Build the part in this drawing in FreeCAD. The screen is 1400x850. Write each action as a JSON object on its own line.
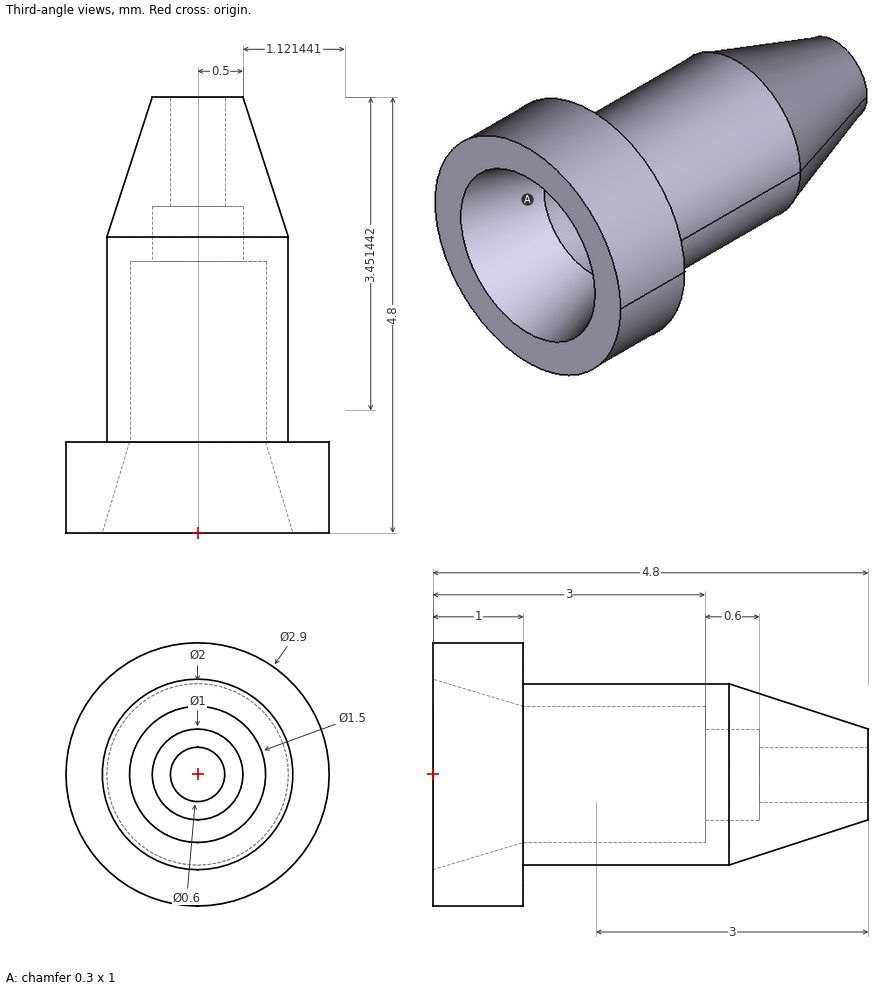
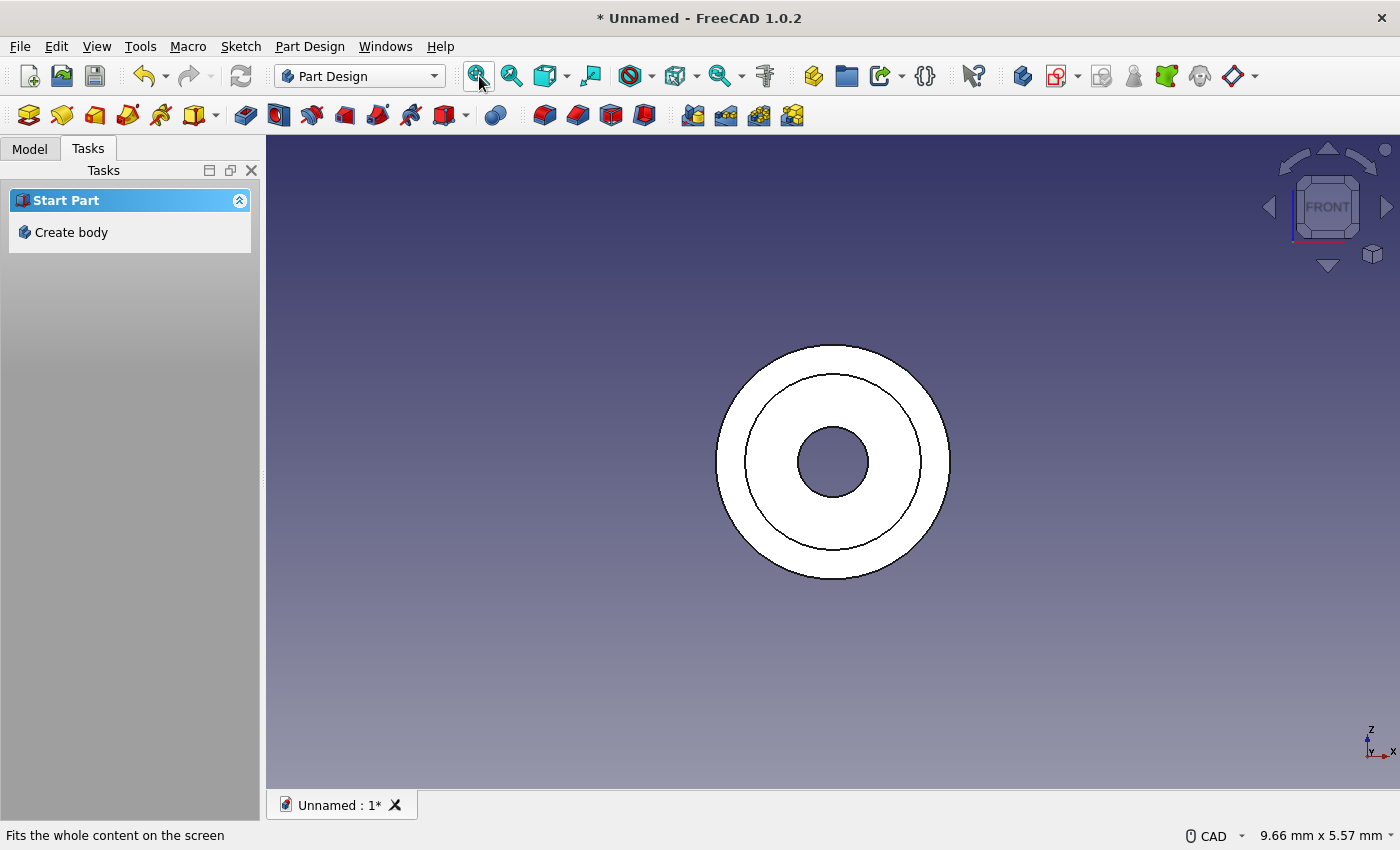
{"action": "left_click", "coordinate": [808, 511]}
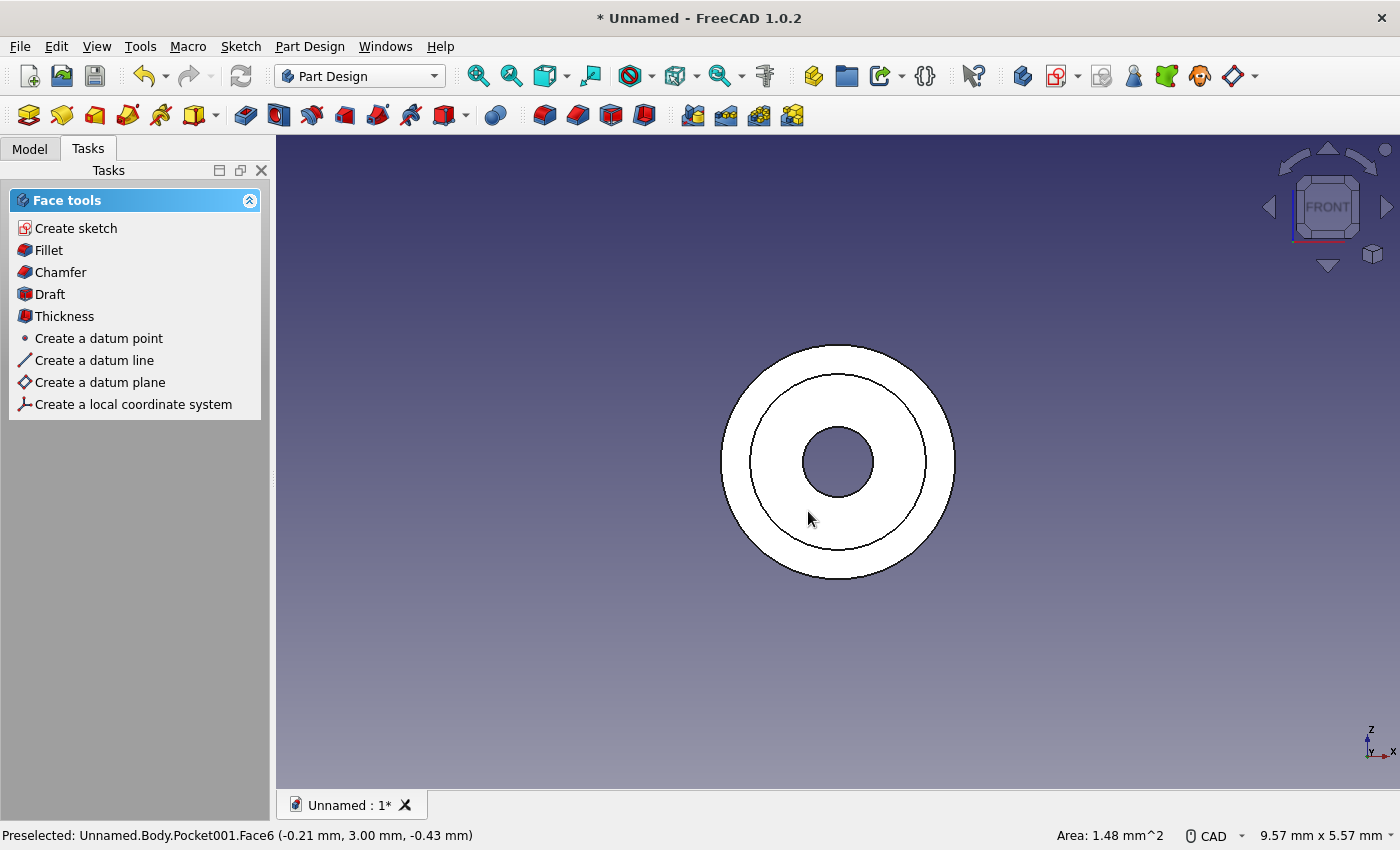
{"action": "left_click", "coordinate": [1056, 76]}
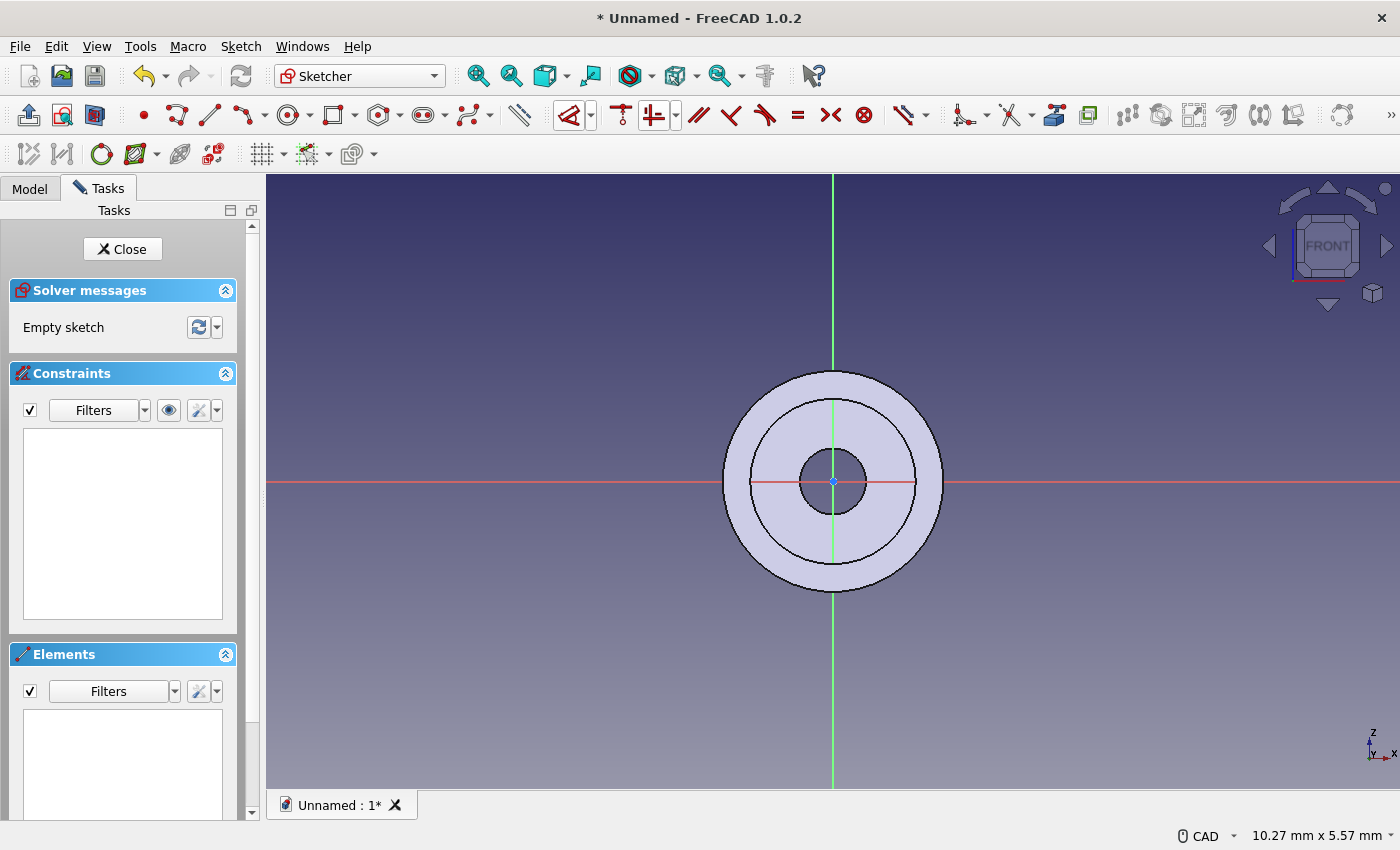
{"action": "key", "text": "q s"}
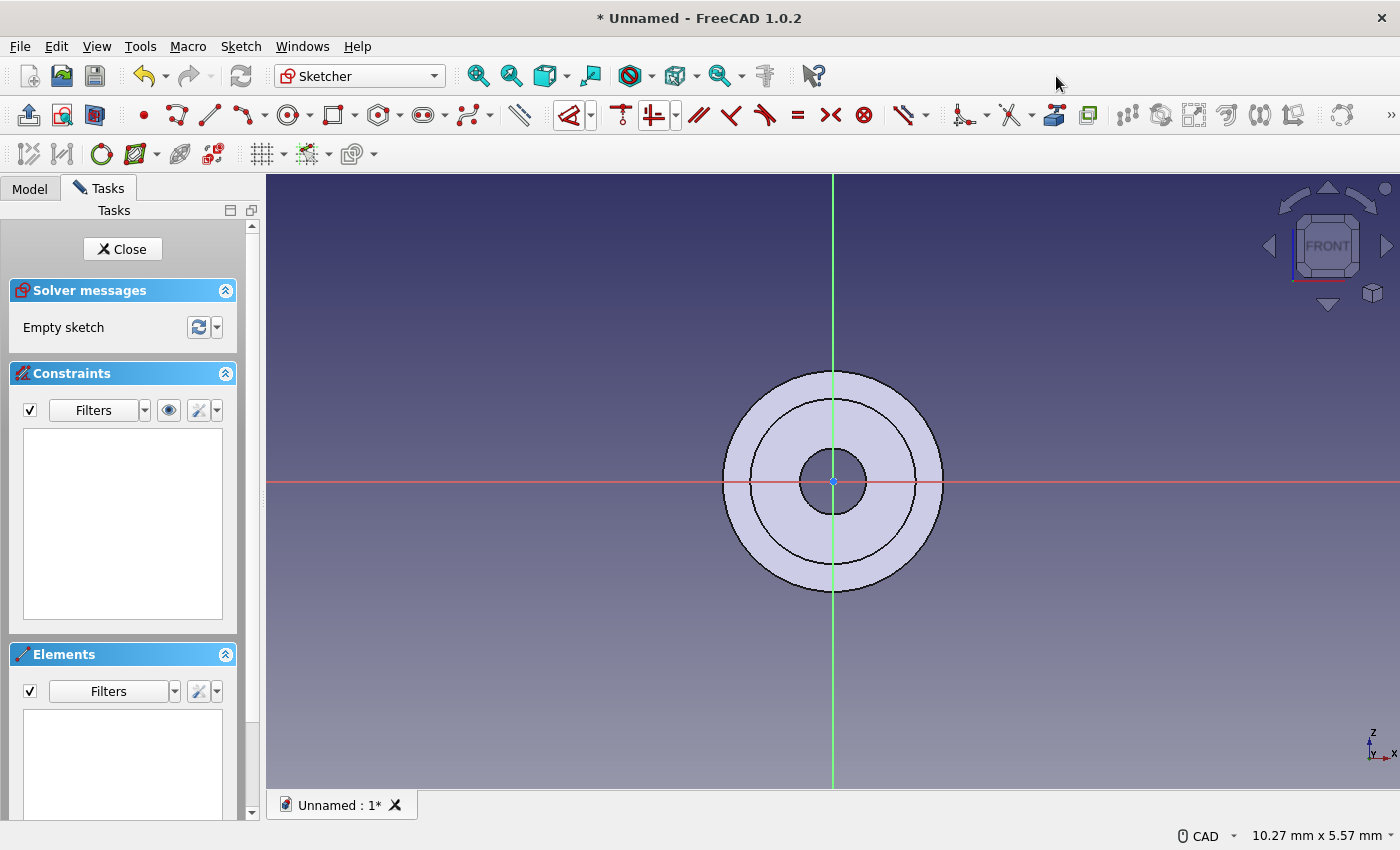
{"action": "scroll", "coordinate": [863, 482], "scroll_direction": "up", "scroll_amount": 6}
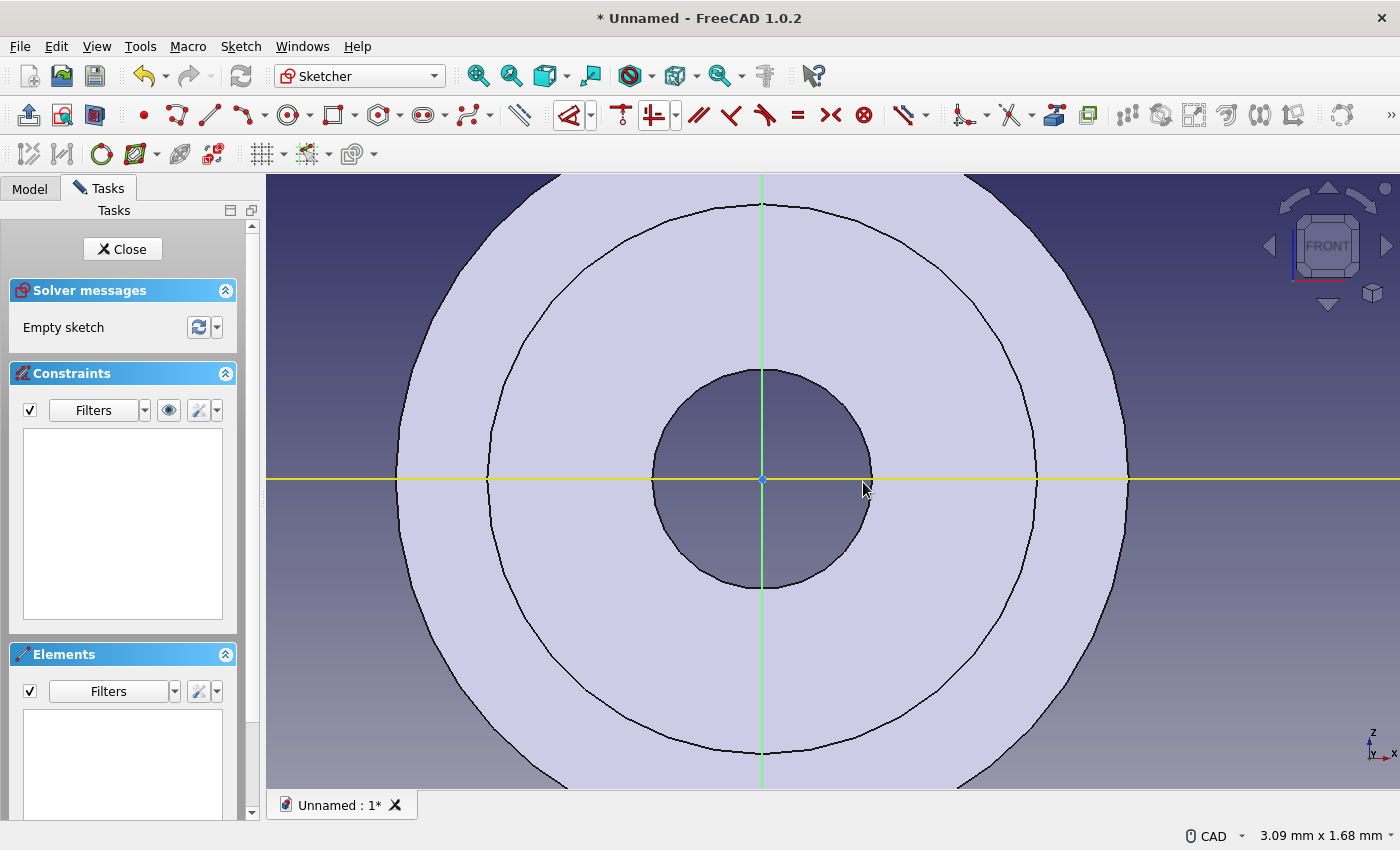
{"action": "left_click", "coordinate": [288, 116]}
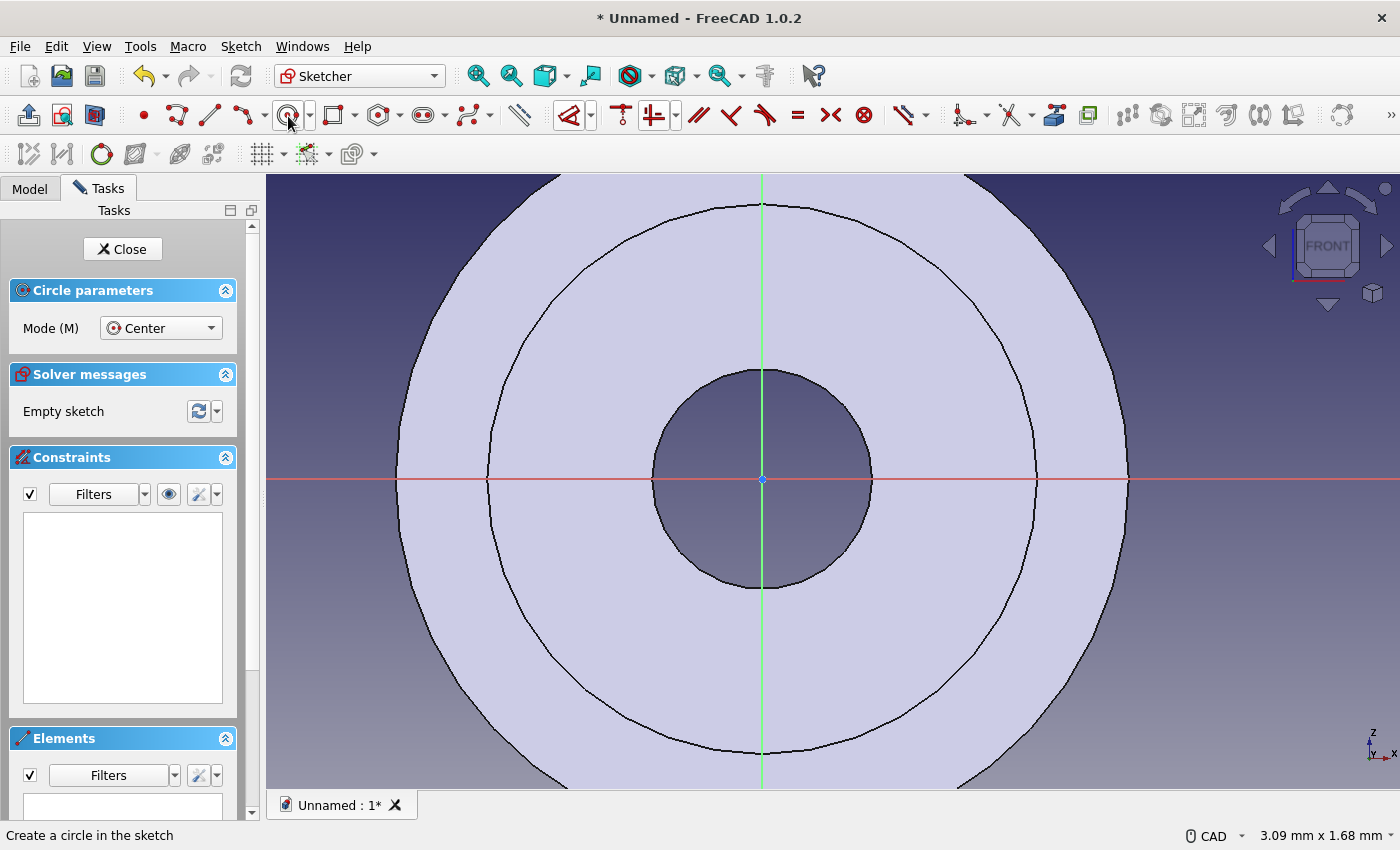
{"action": "left_click", "coordinate": [762, 479]}
{"action": "left_click", "coordinate": [892, 350]}
{"action": "key", "text": "Escape"}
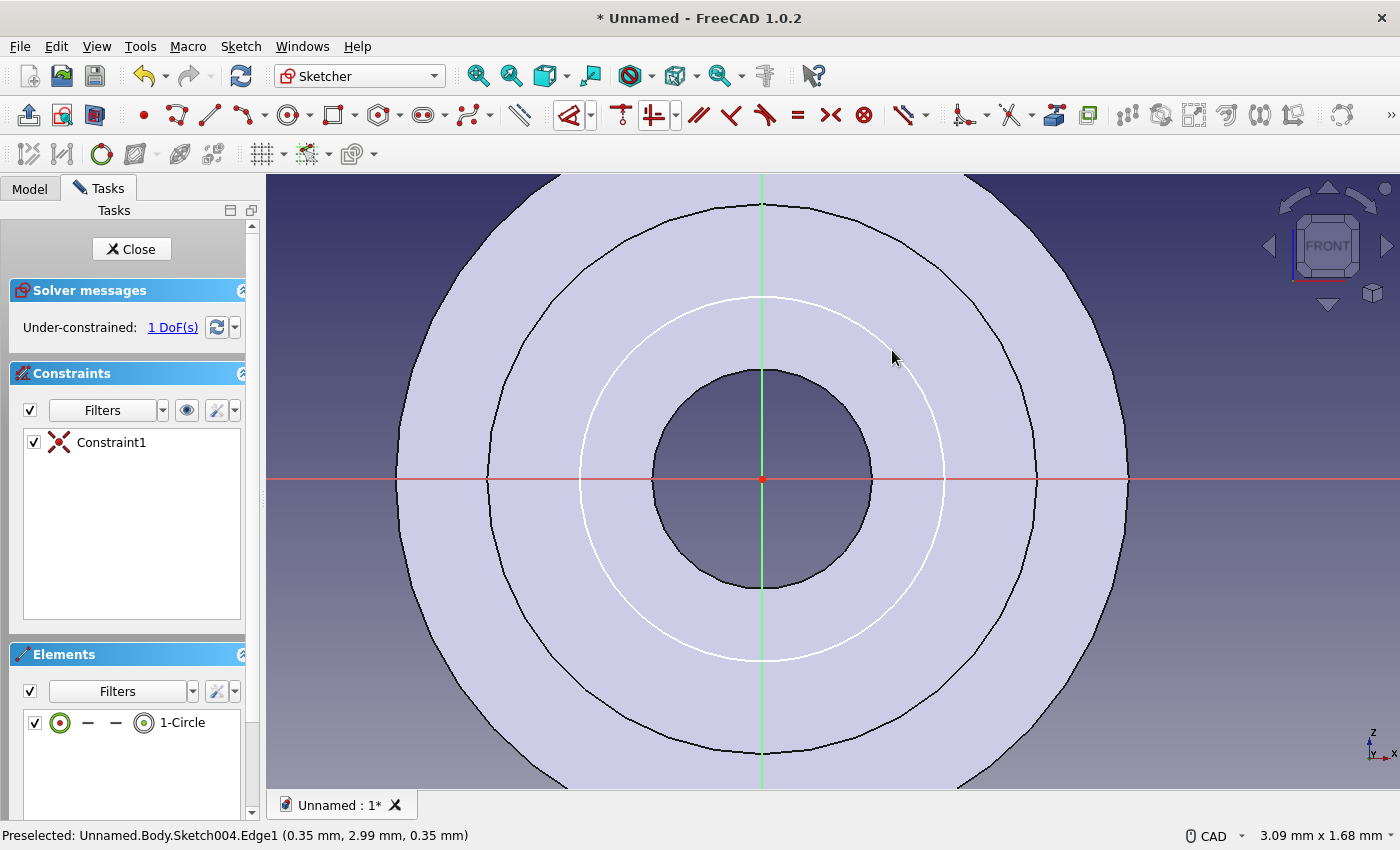
{"action": "left_click", "coordinate": [891, 350]}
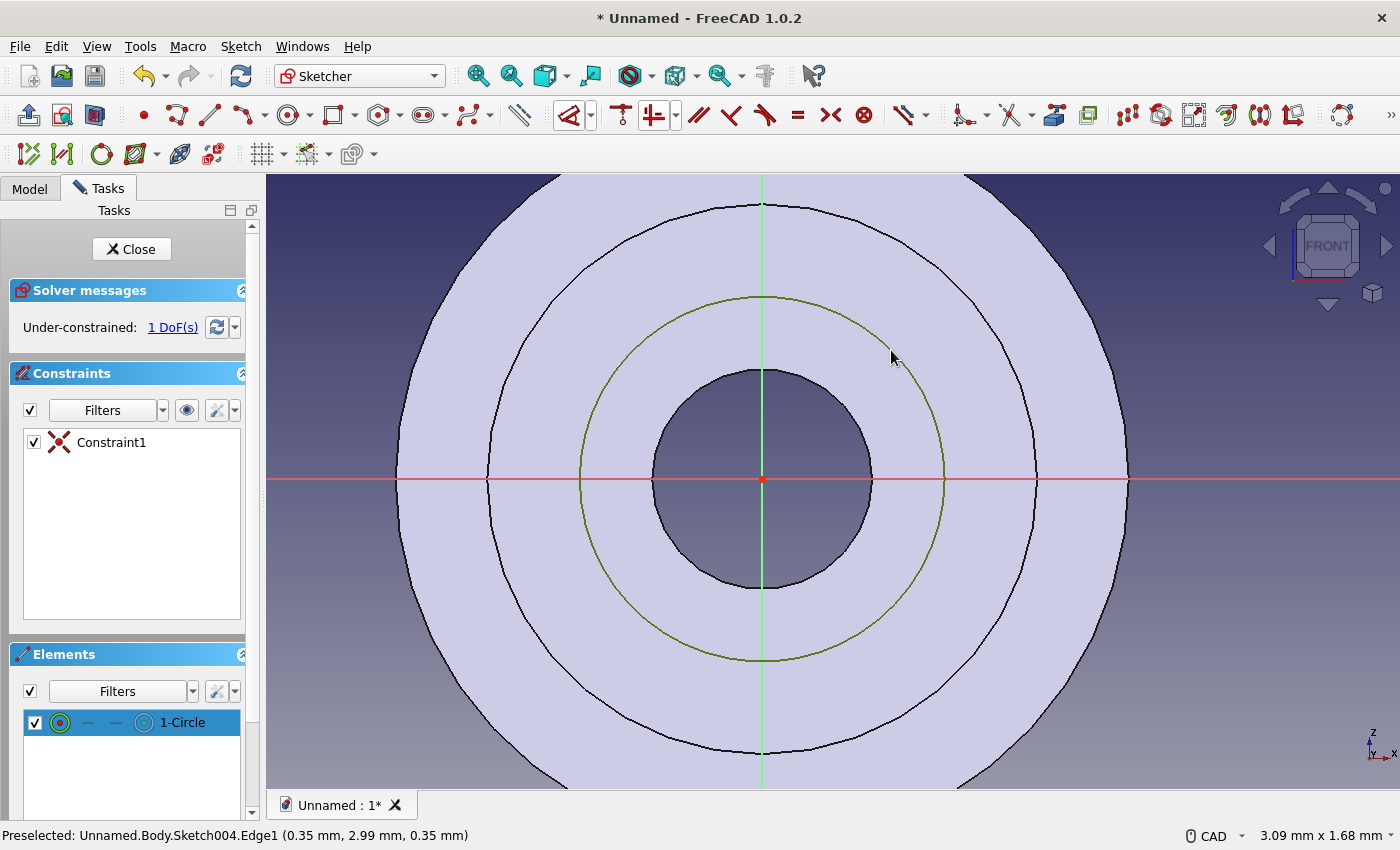
{"action": "key", "text": "k o"}